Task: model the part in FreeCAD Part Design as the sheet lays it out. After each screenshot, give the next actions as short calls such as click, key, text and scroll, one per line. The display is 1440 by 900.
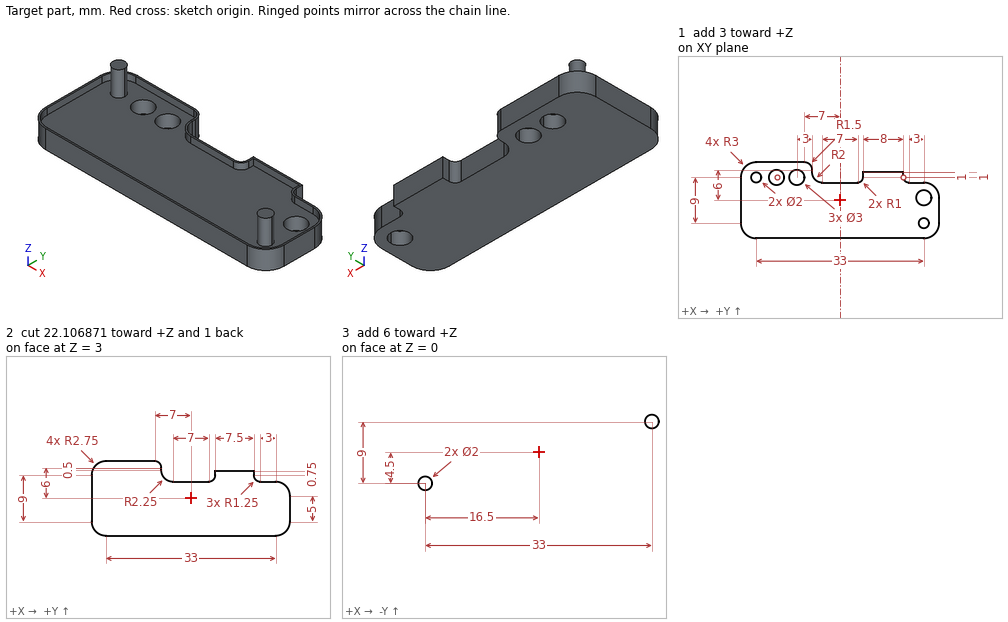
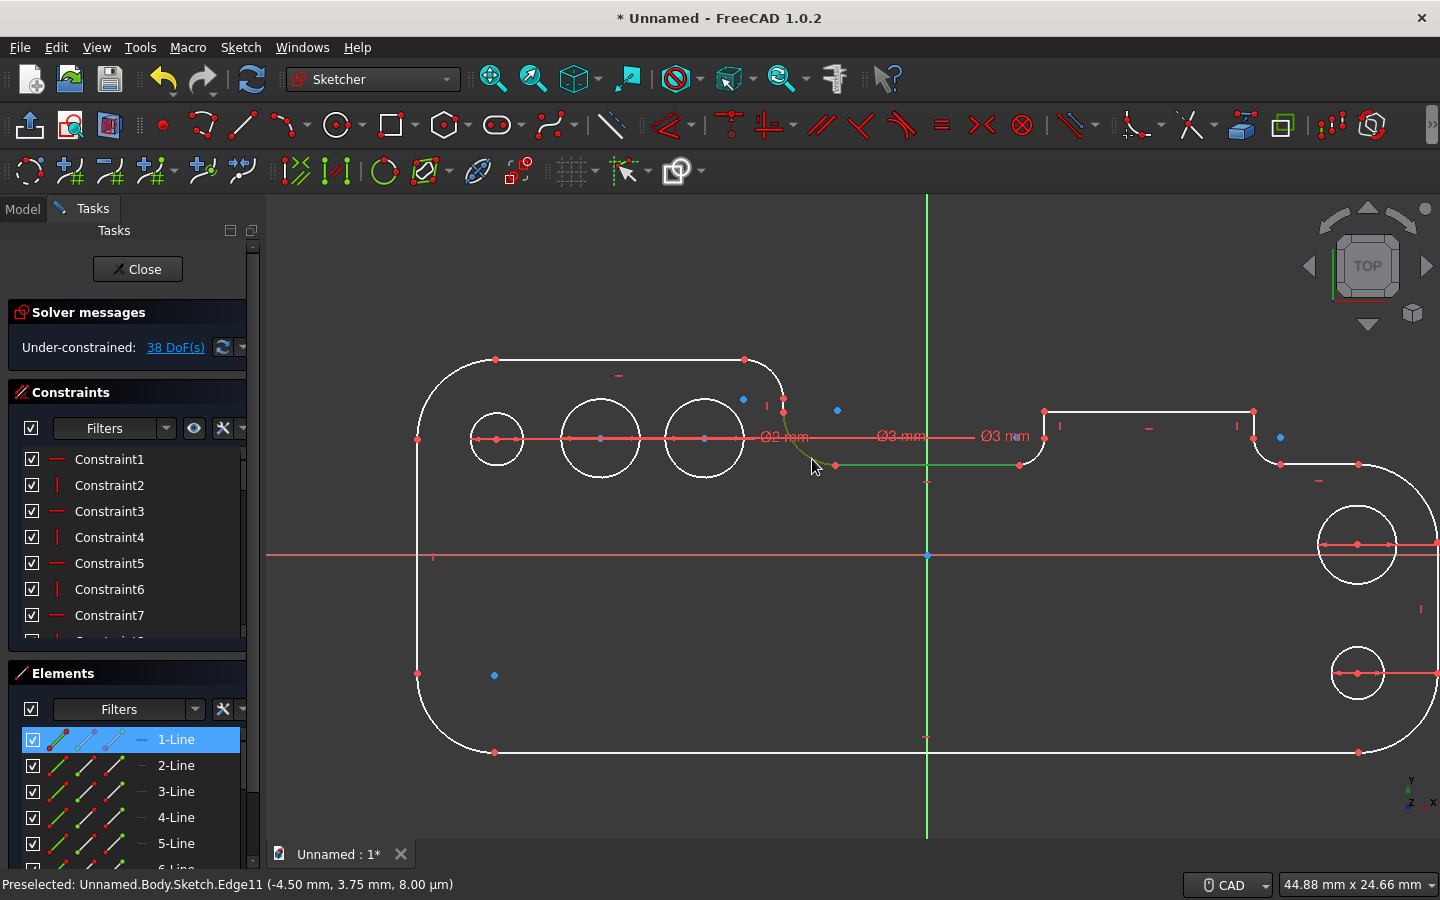
click(902, 126)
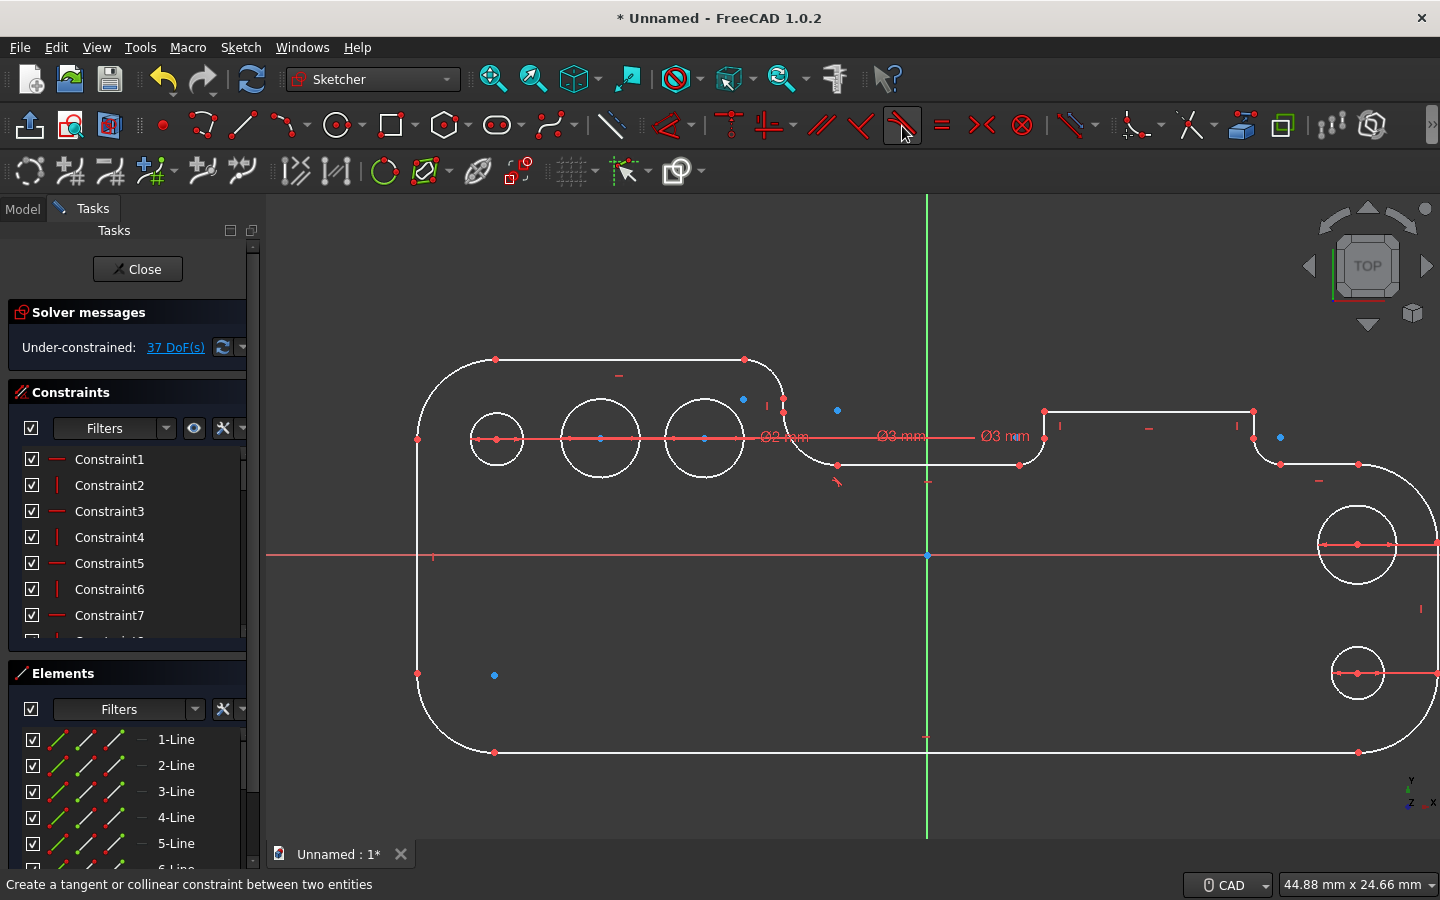
click(965, 465)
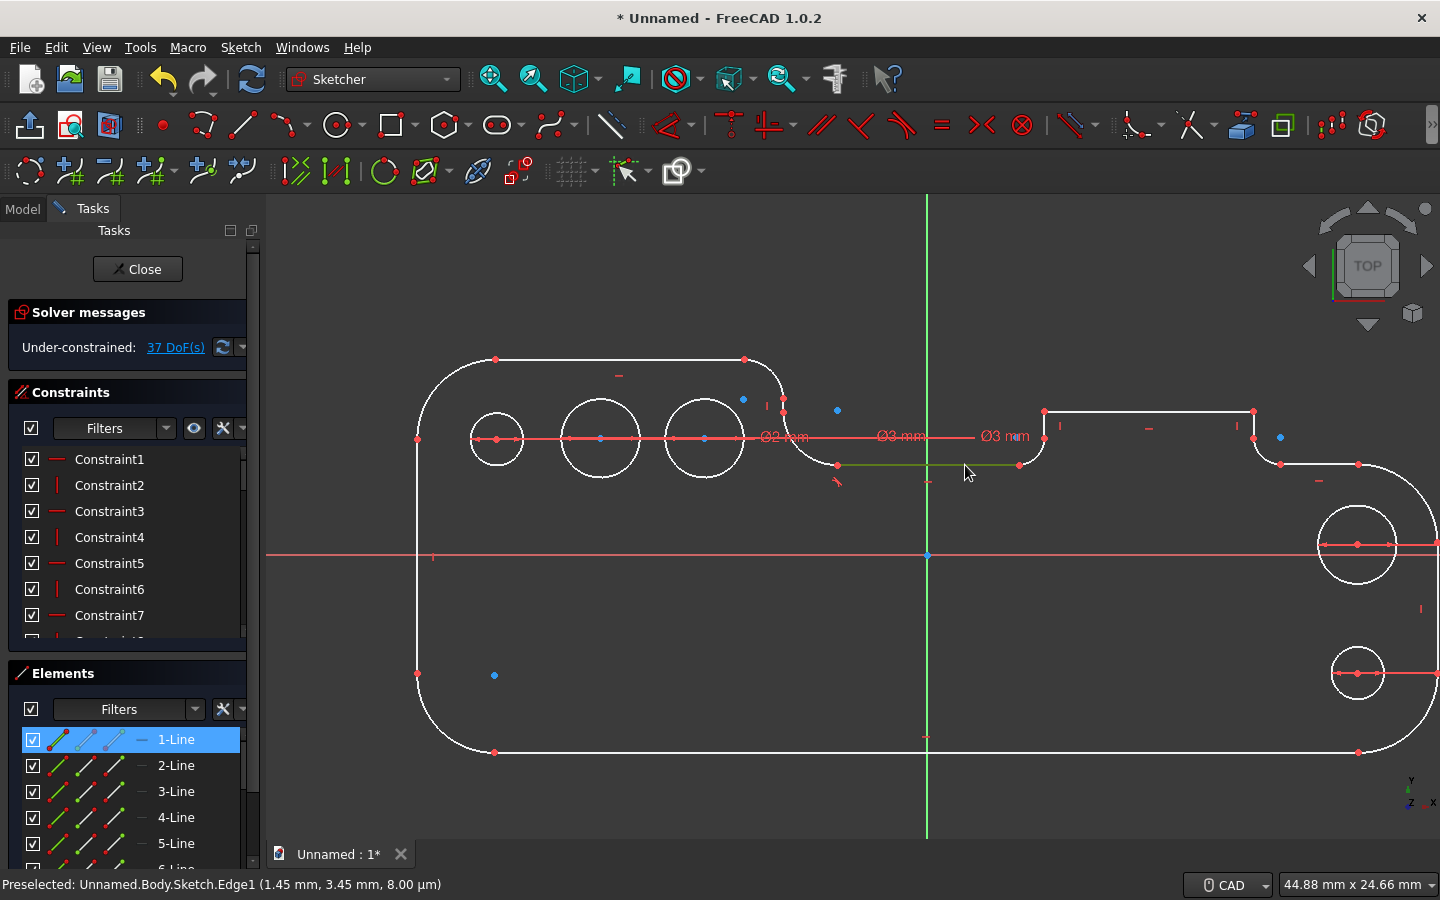
click(1031, 462)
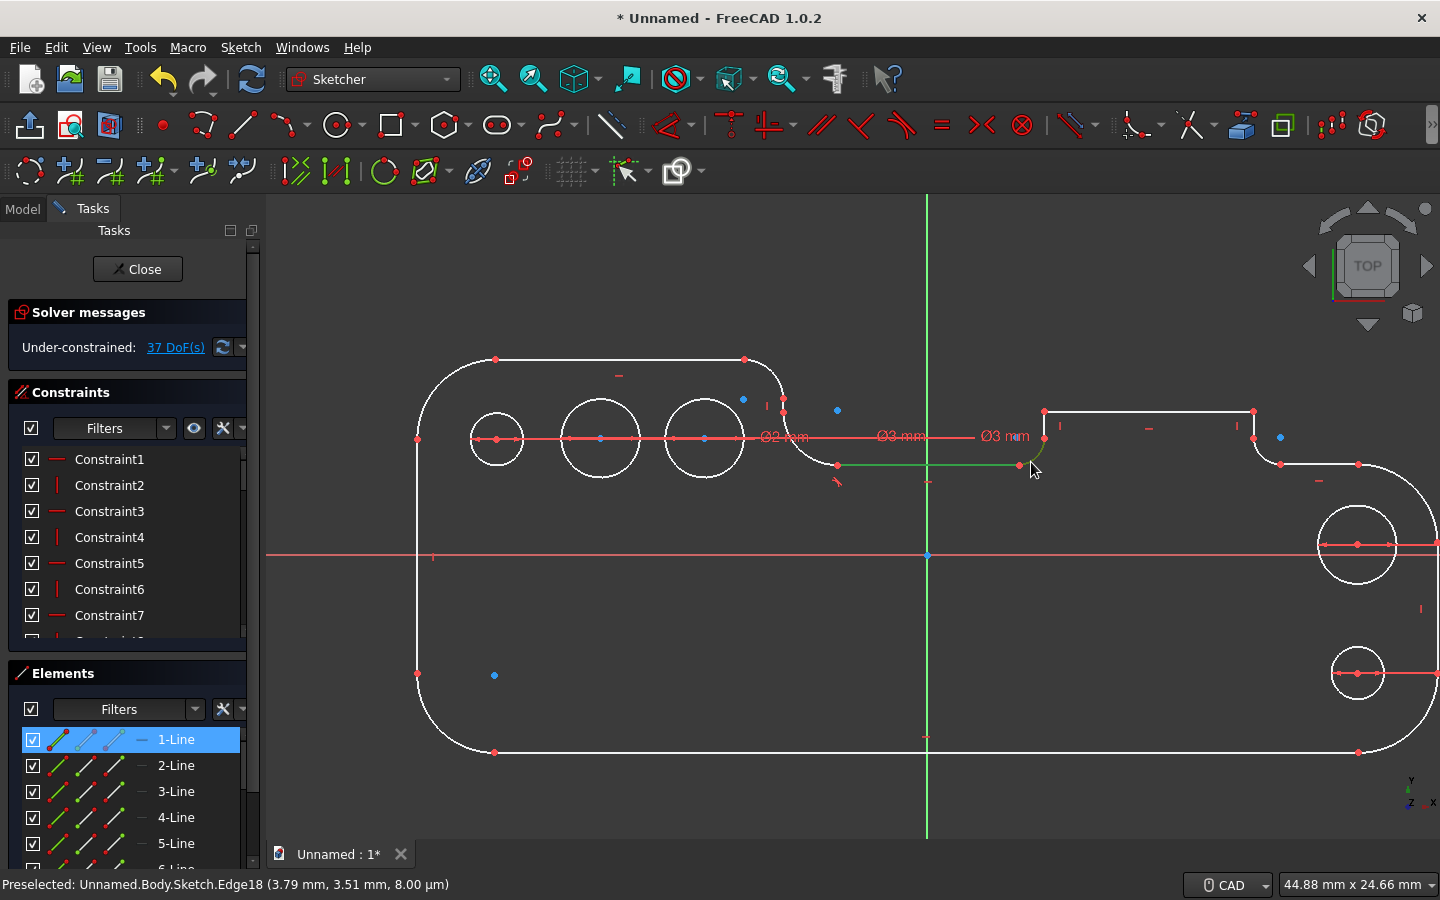
click(902, 126)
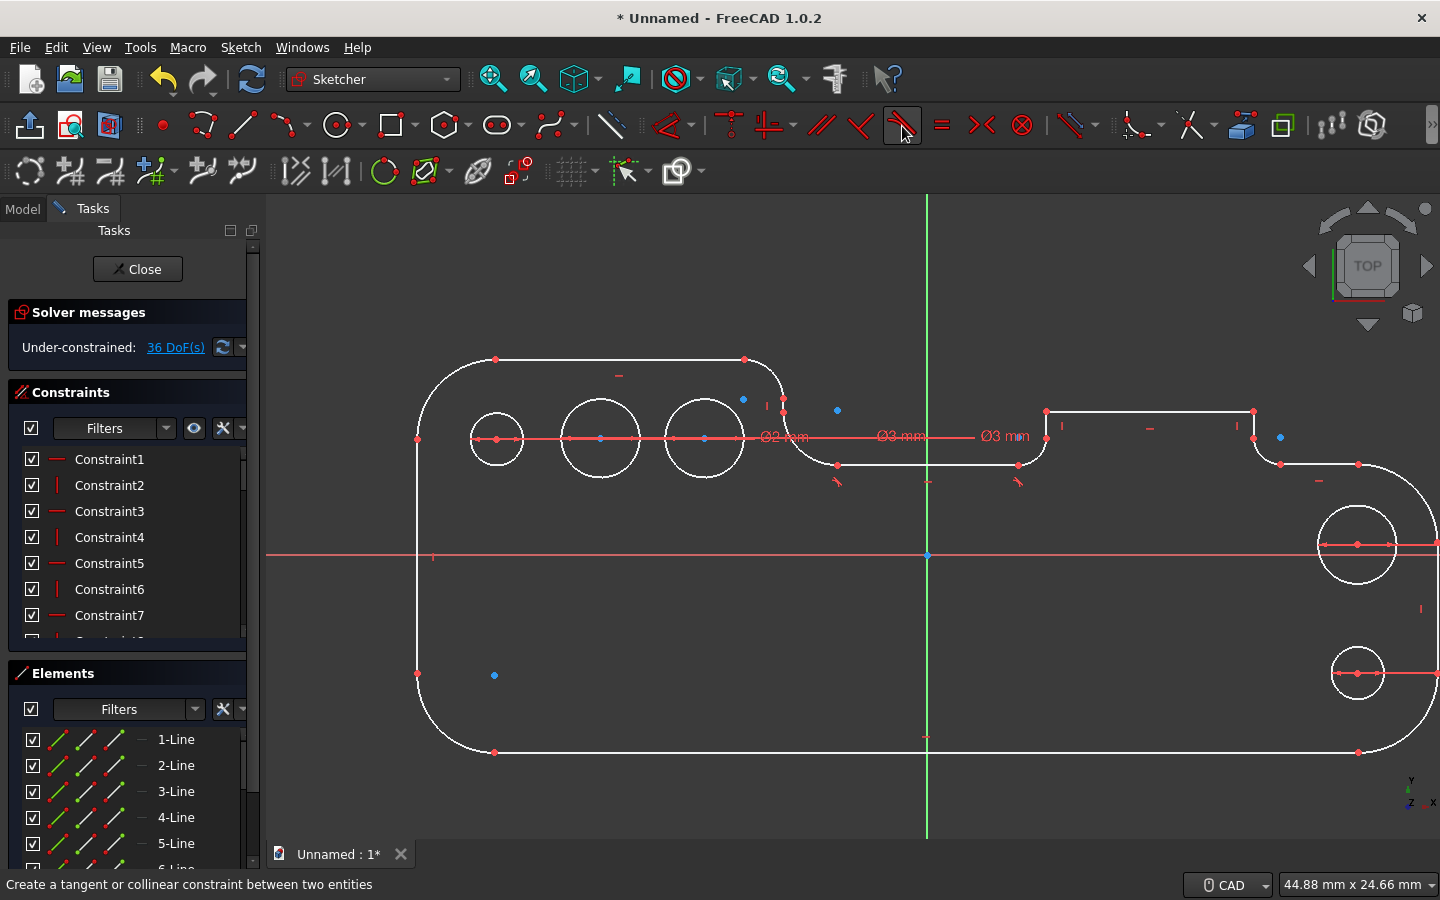
scroll(783, 406, up, 4)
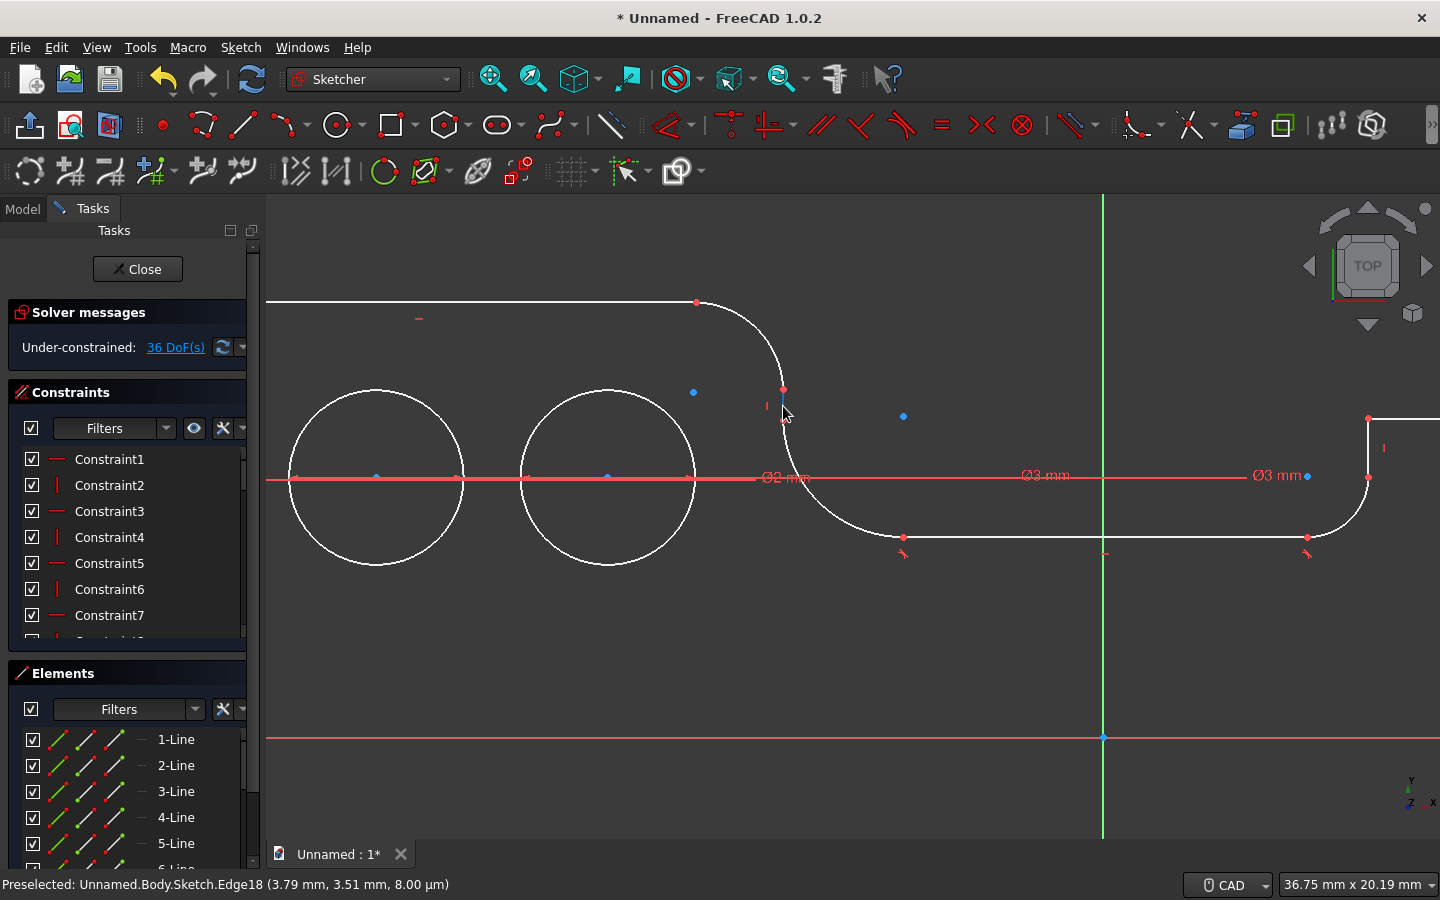
click(783, 405)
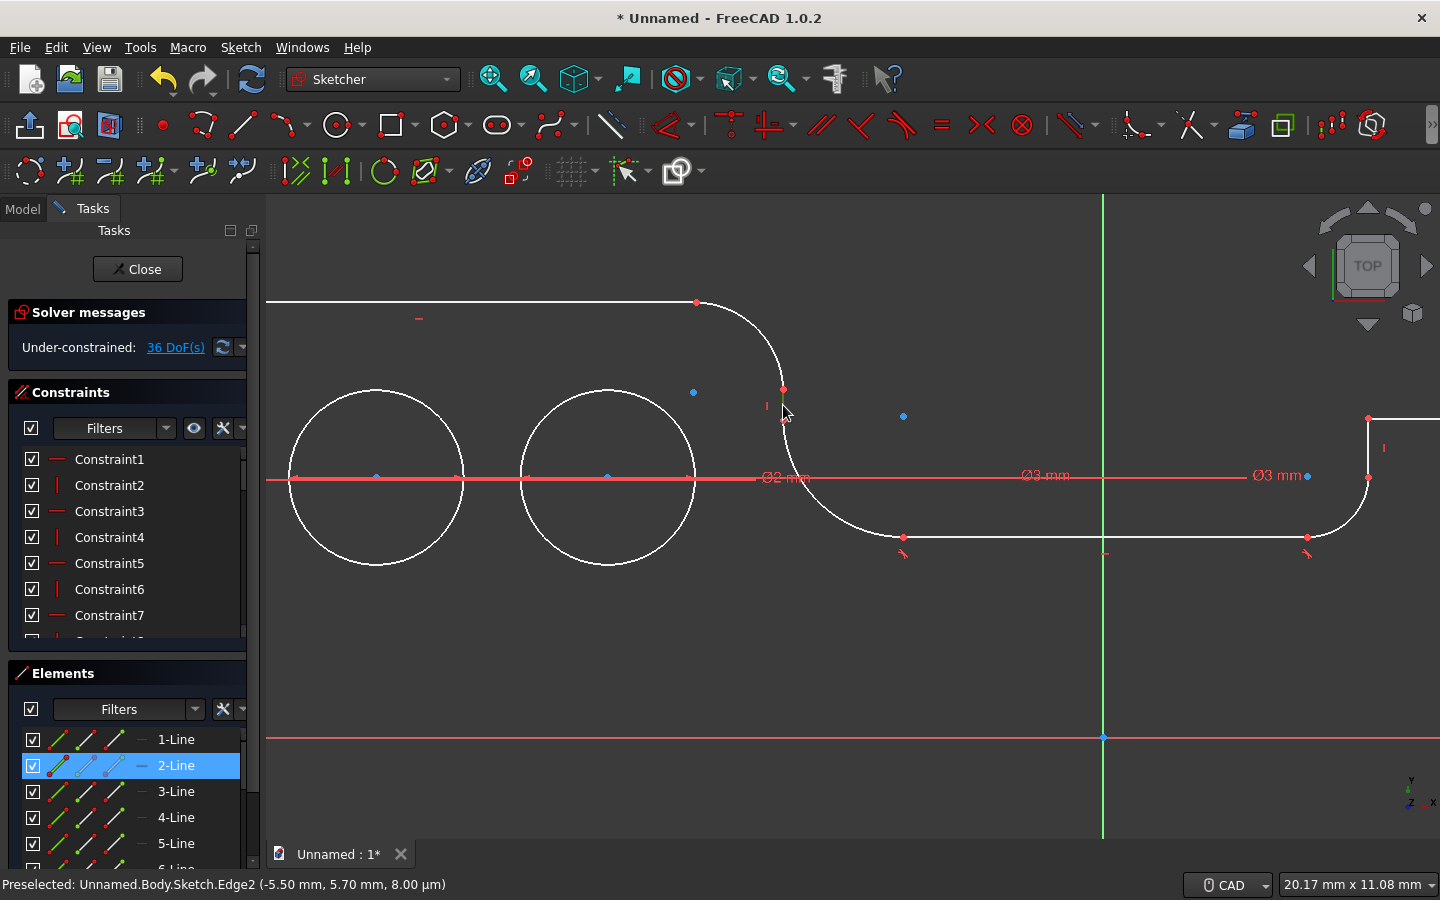
click(850, 525)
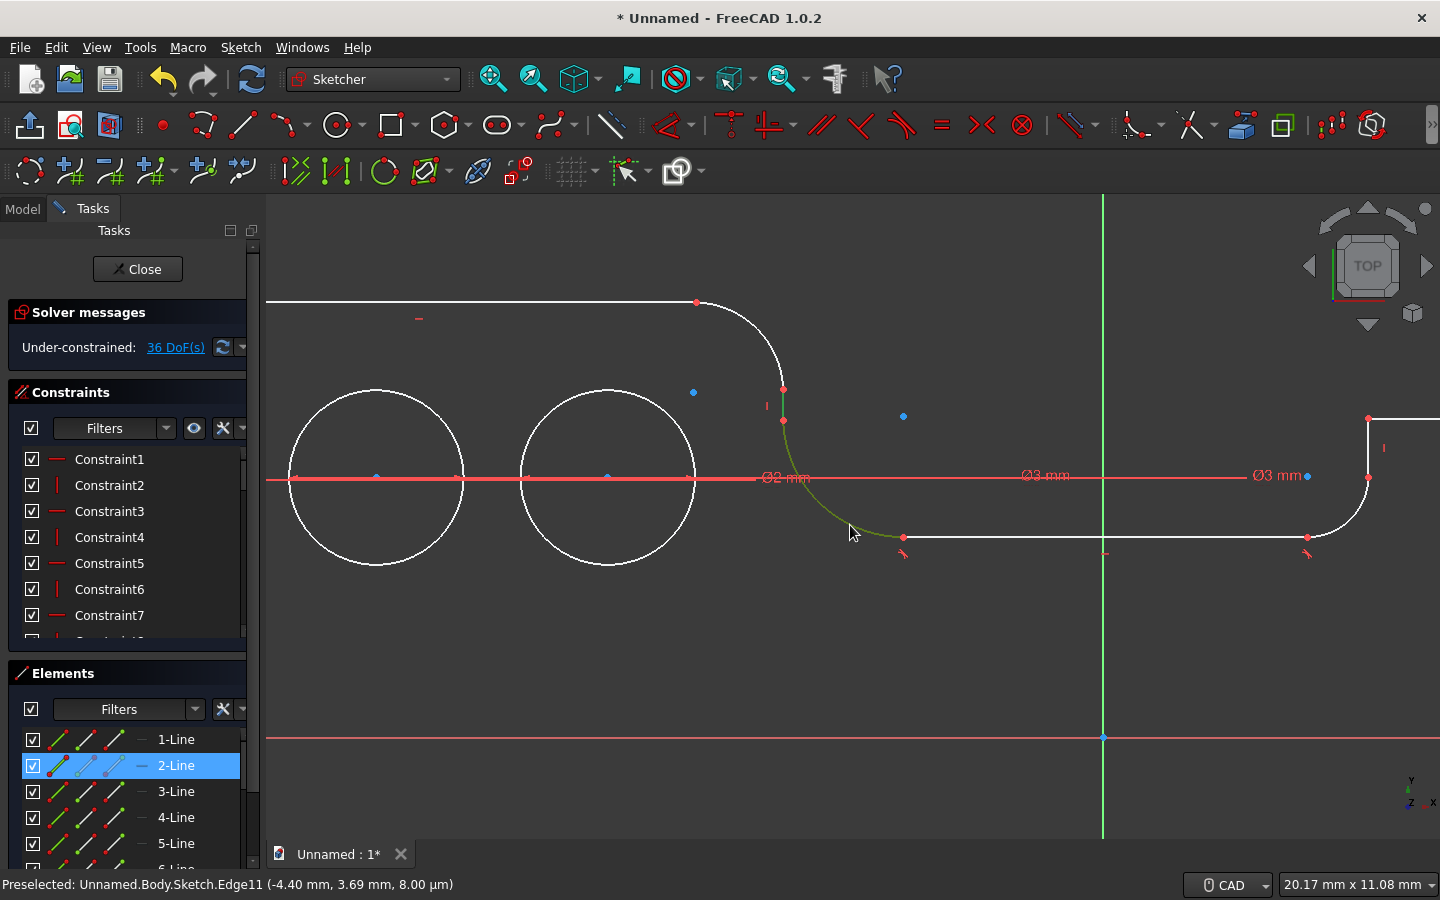
key(t)